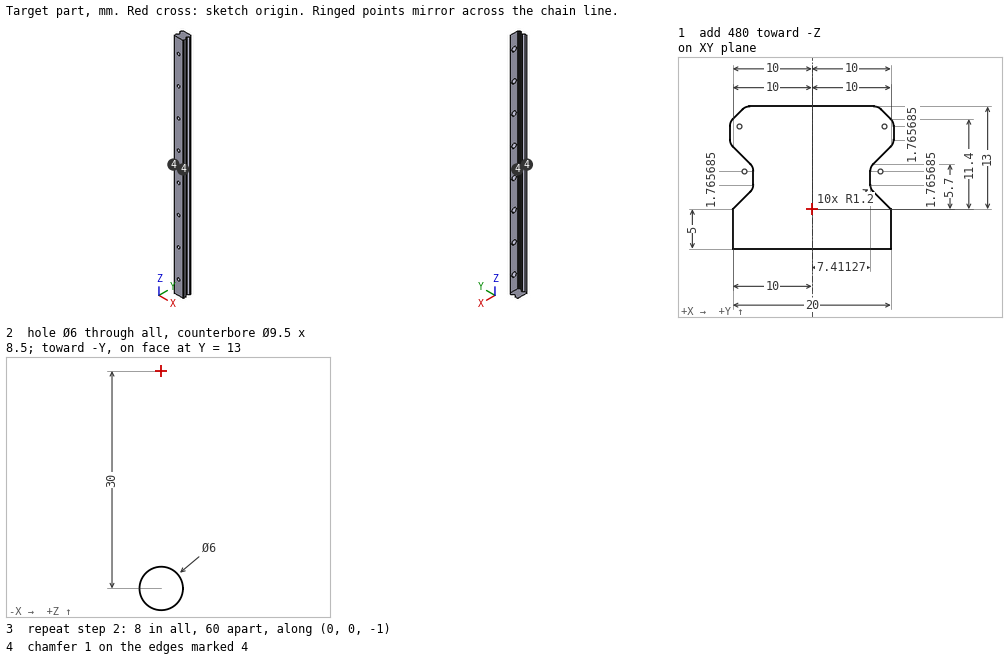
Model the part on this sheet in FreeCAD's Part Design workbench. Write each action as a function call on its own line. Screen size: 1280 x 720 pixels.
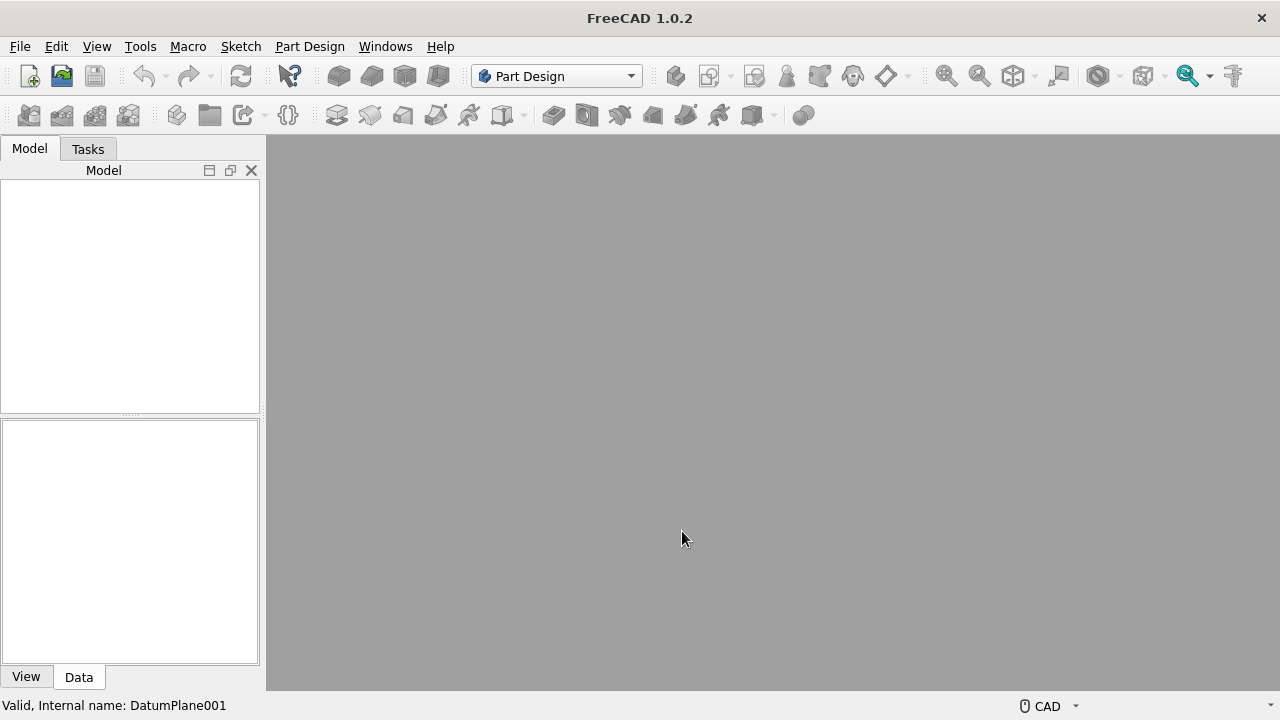
key(ctrl+n)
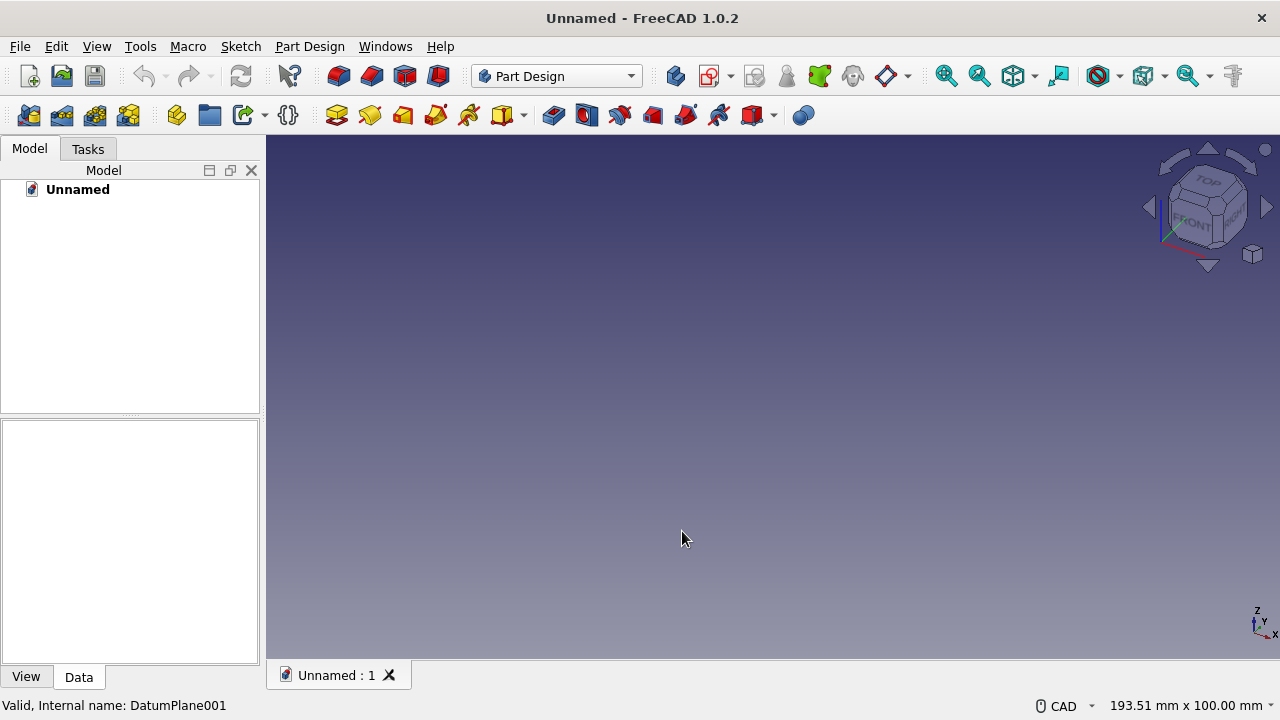
click(708, 76)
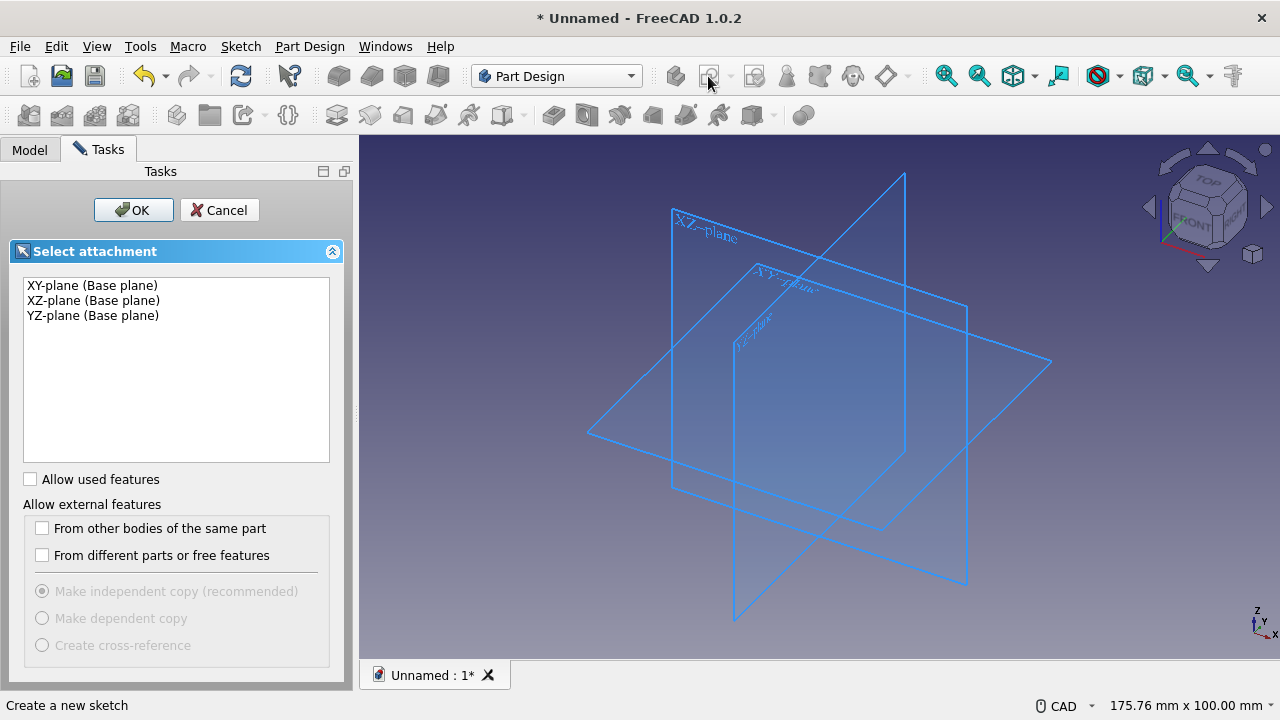
click(84, 286)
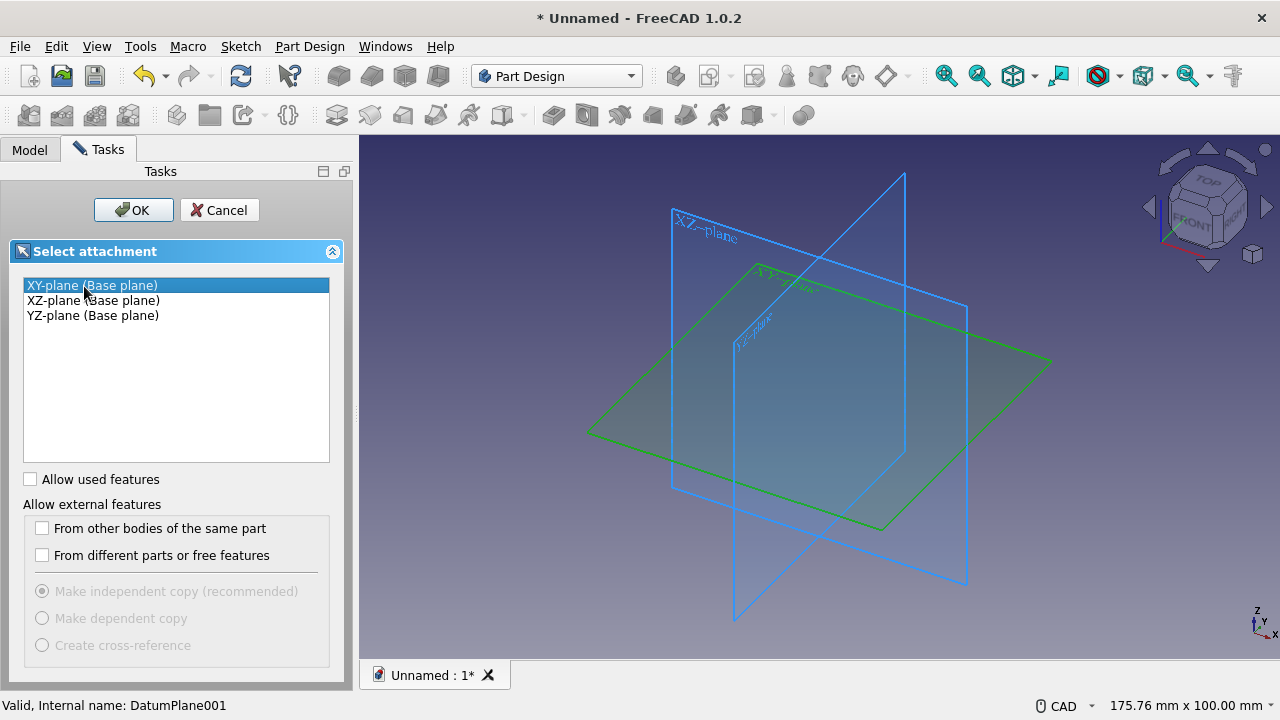
click(134, 210)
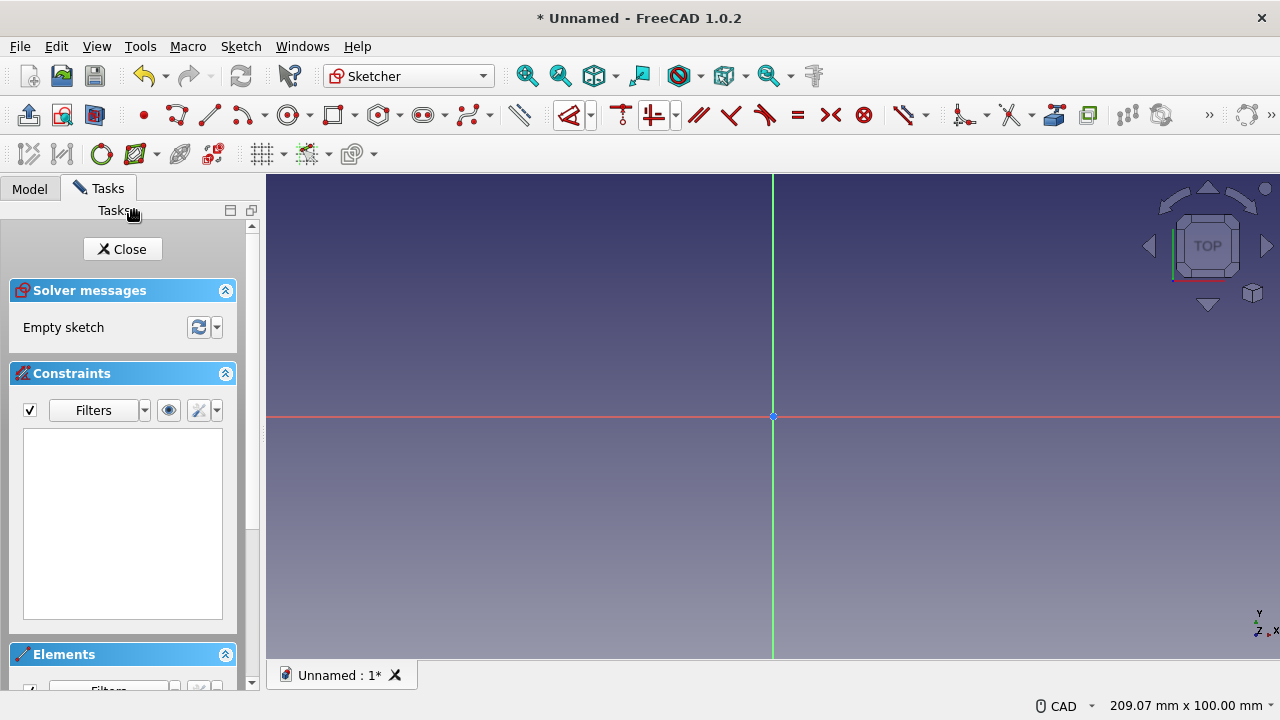
scroll(803, 389, up, 6)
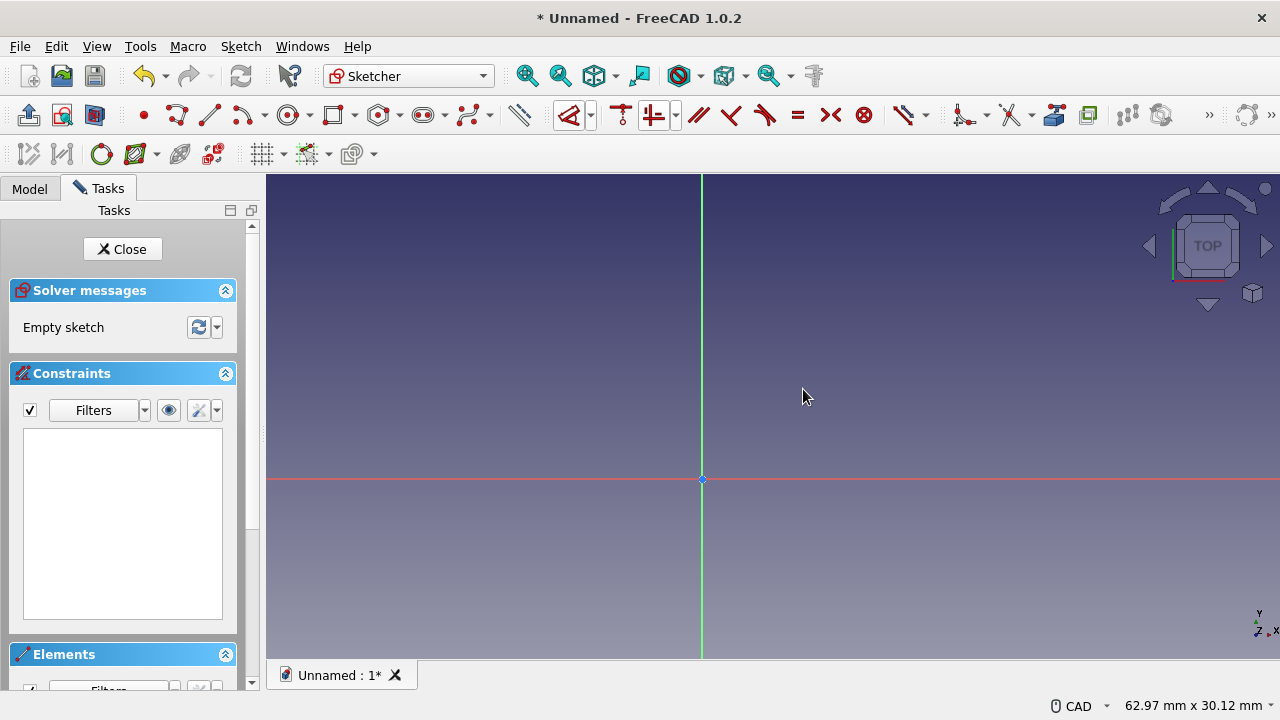
click(210, 116)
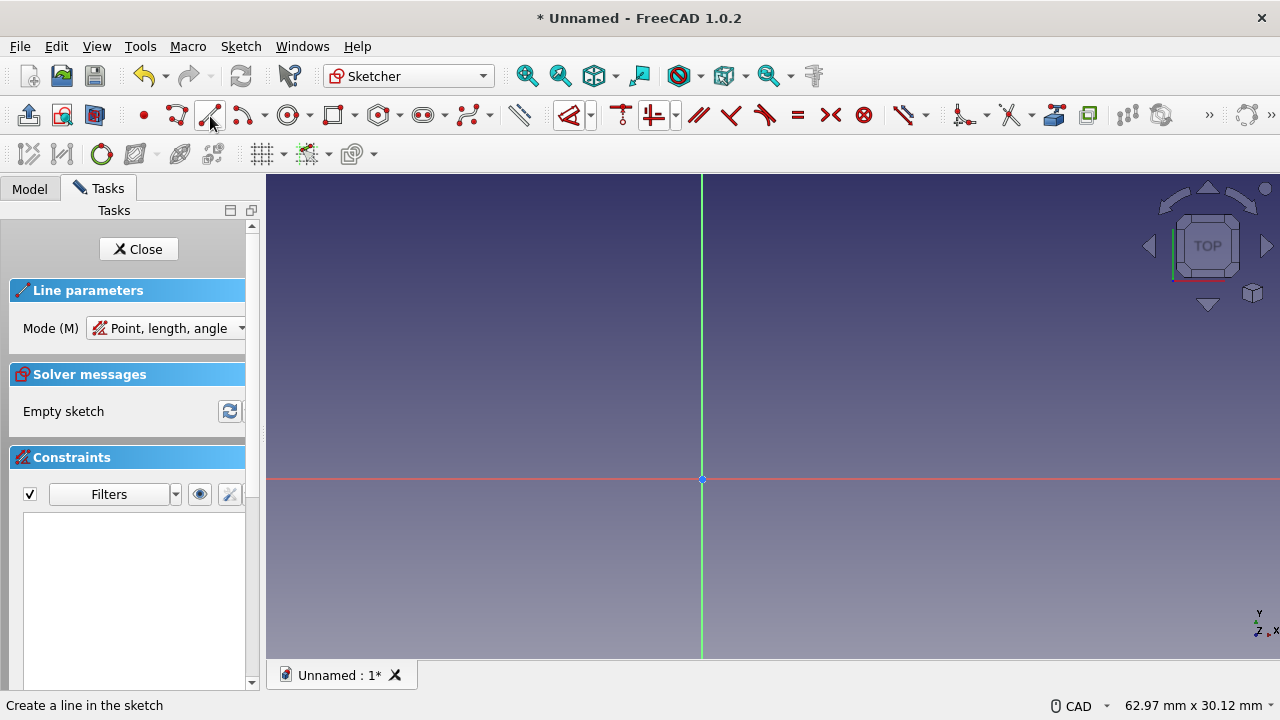
click(822, 430)
click(822, 401)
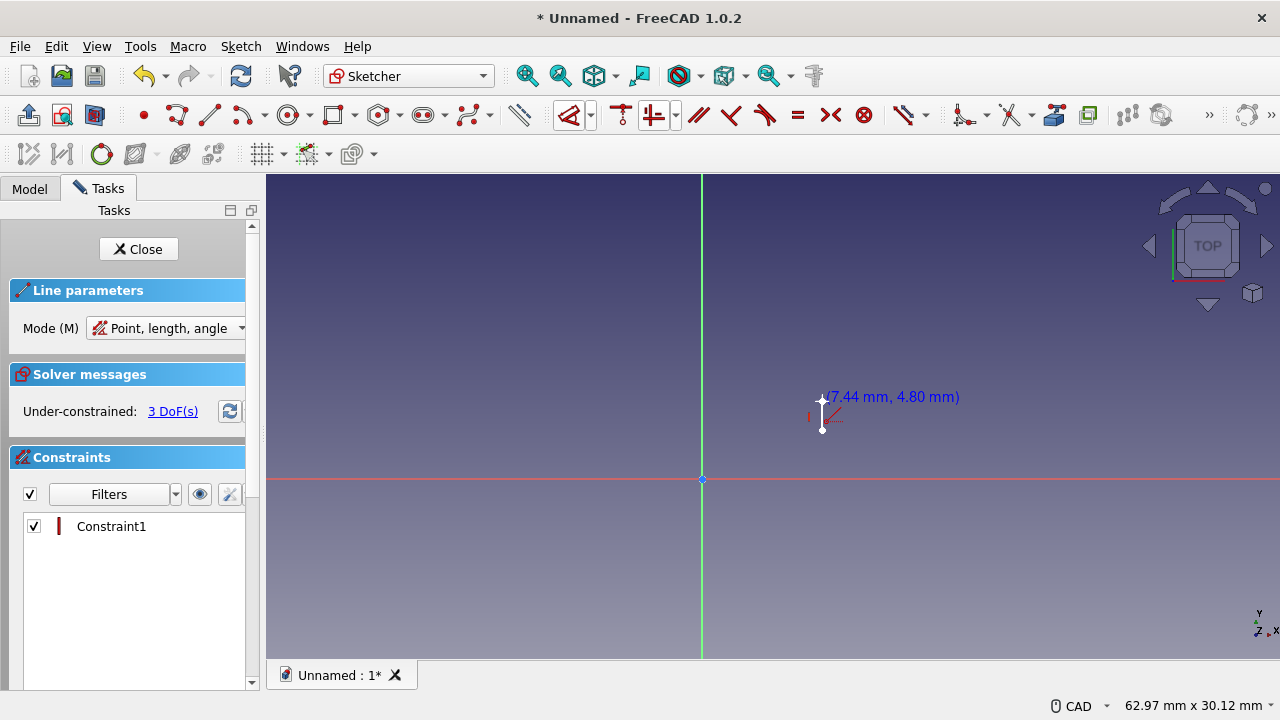
click(827, 387)
click(863, 351)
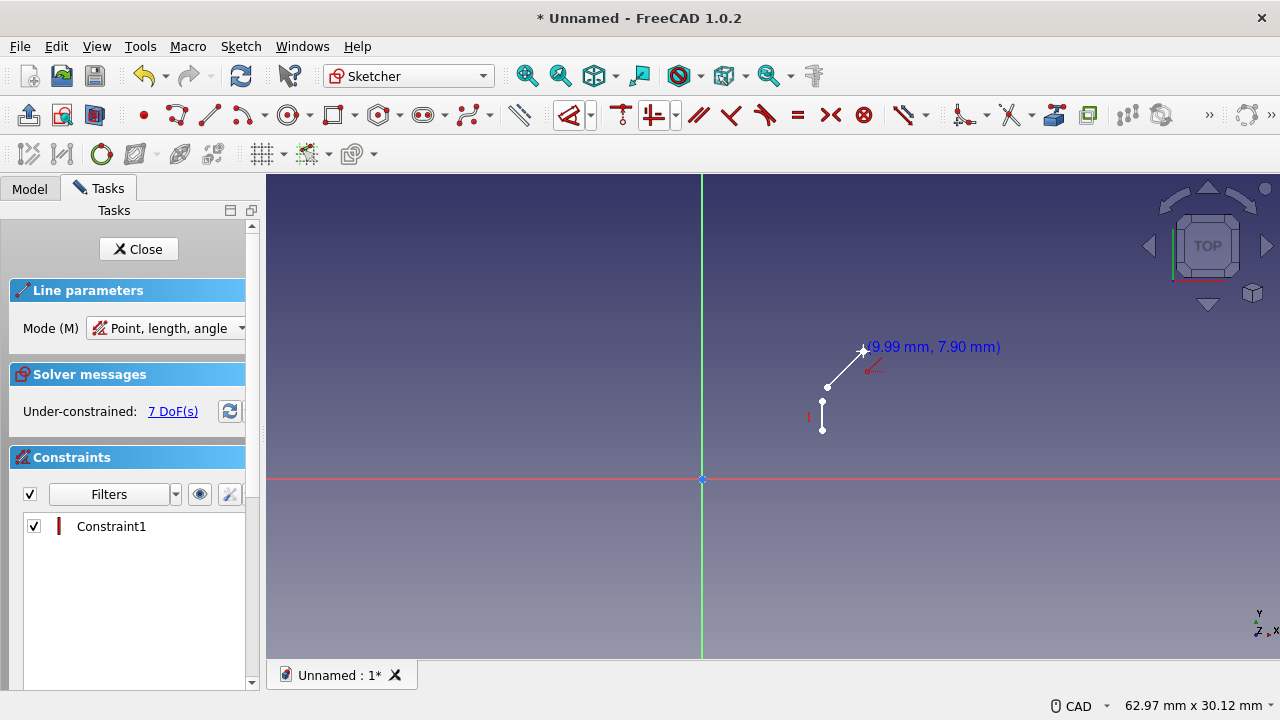
click(869, 338)
click(869, 309)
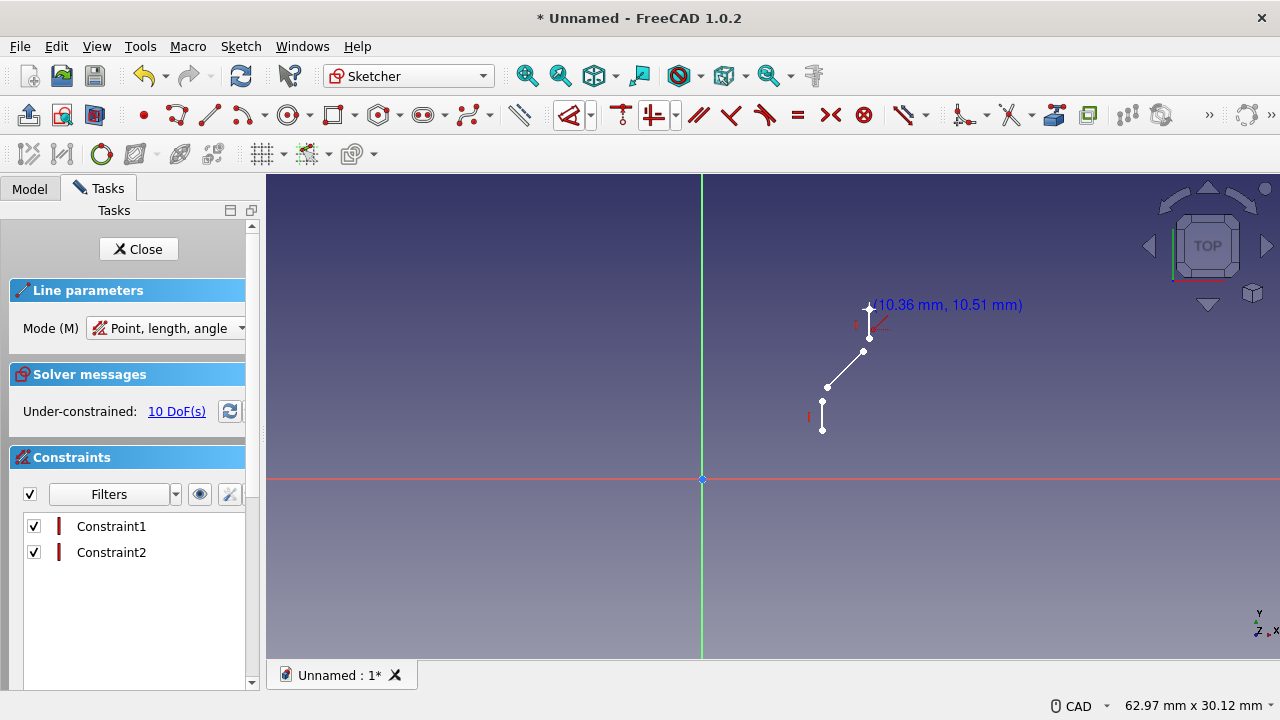
click(863, 296)
click(843, 276)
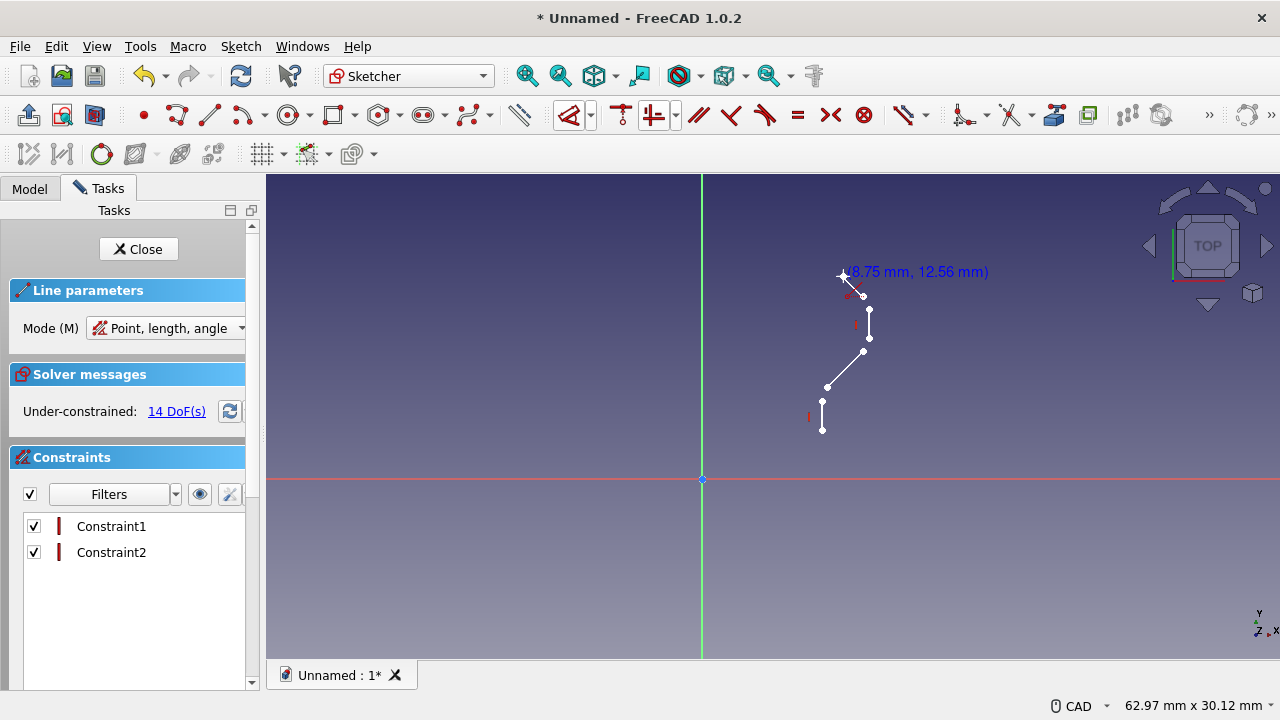
click(829, 270)
click(575, 270)